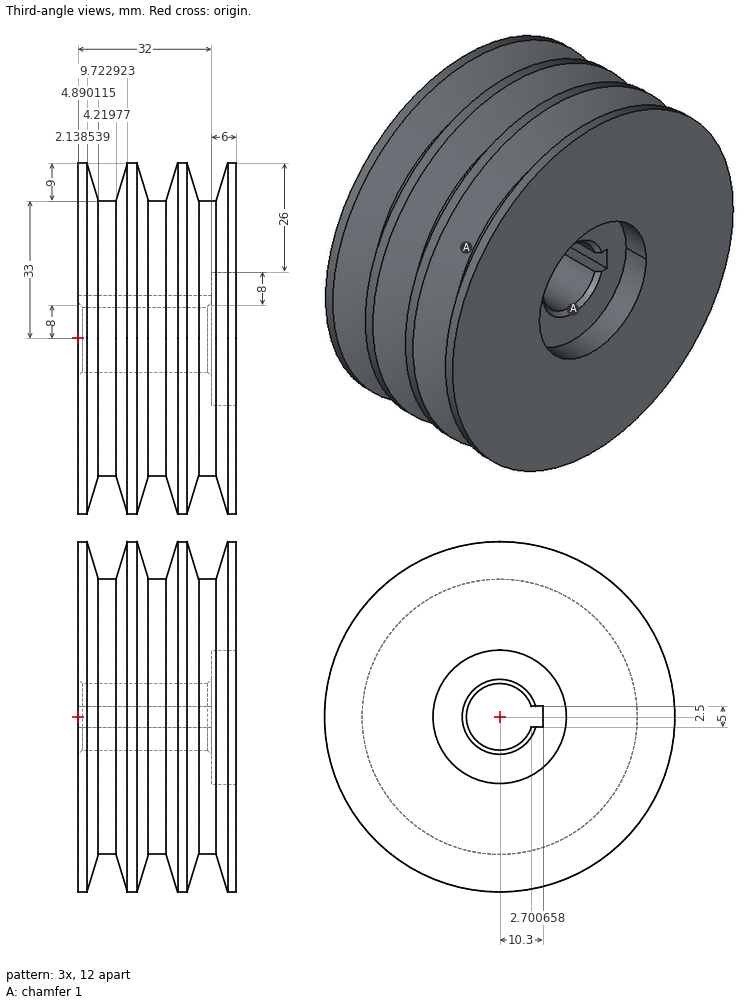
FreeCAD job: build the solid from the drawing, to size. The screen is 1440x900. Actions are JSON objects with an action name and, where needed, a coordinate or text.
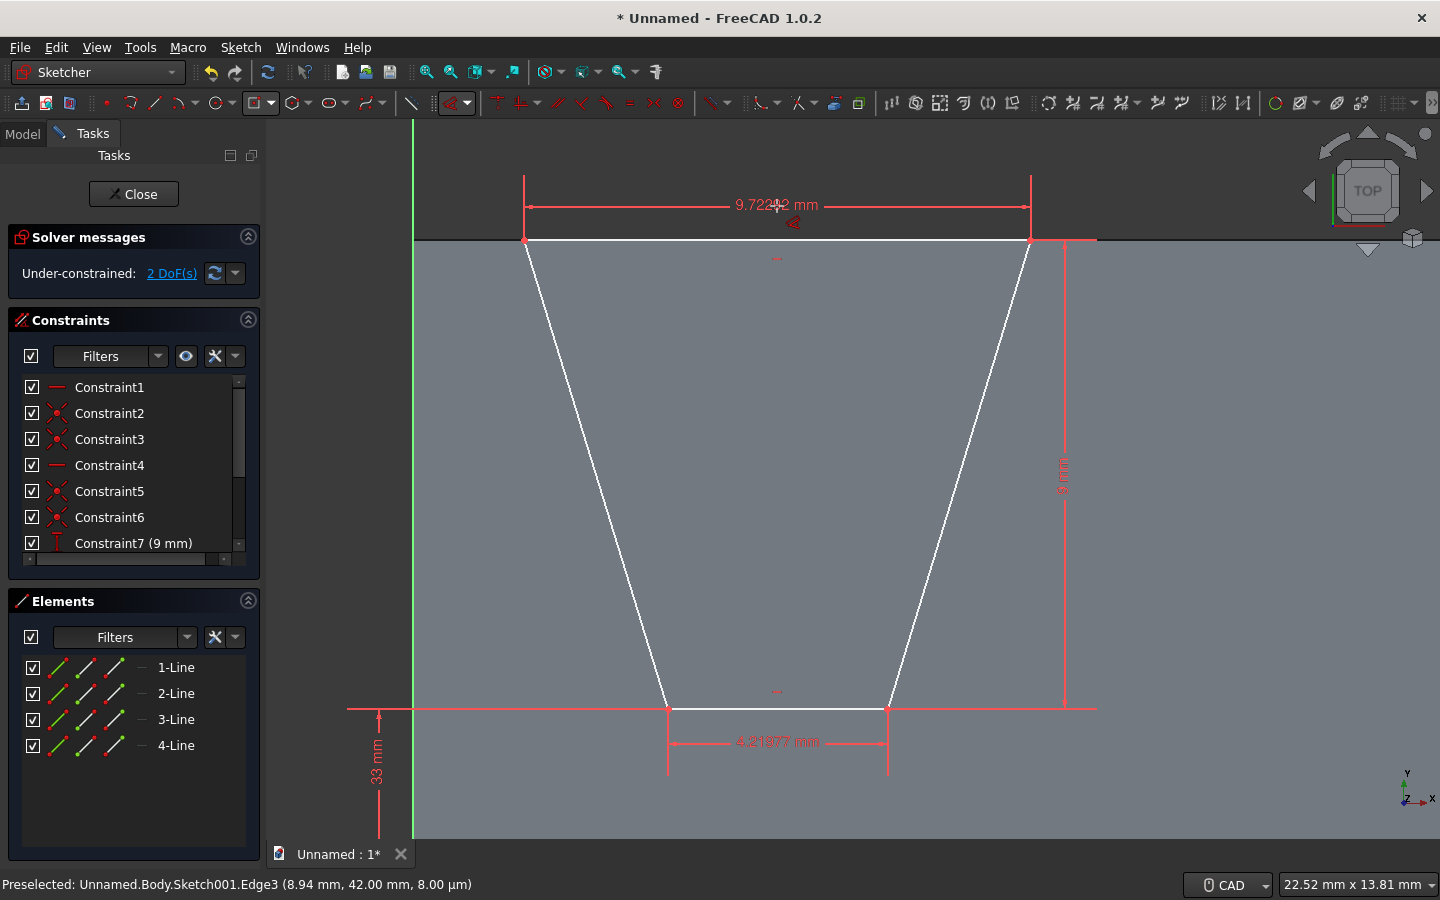
{"action": "left_click", "coordinate": [668, 709]}
{"action": "left_click", "coordinate": [540, 675]}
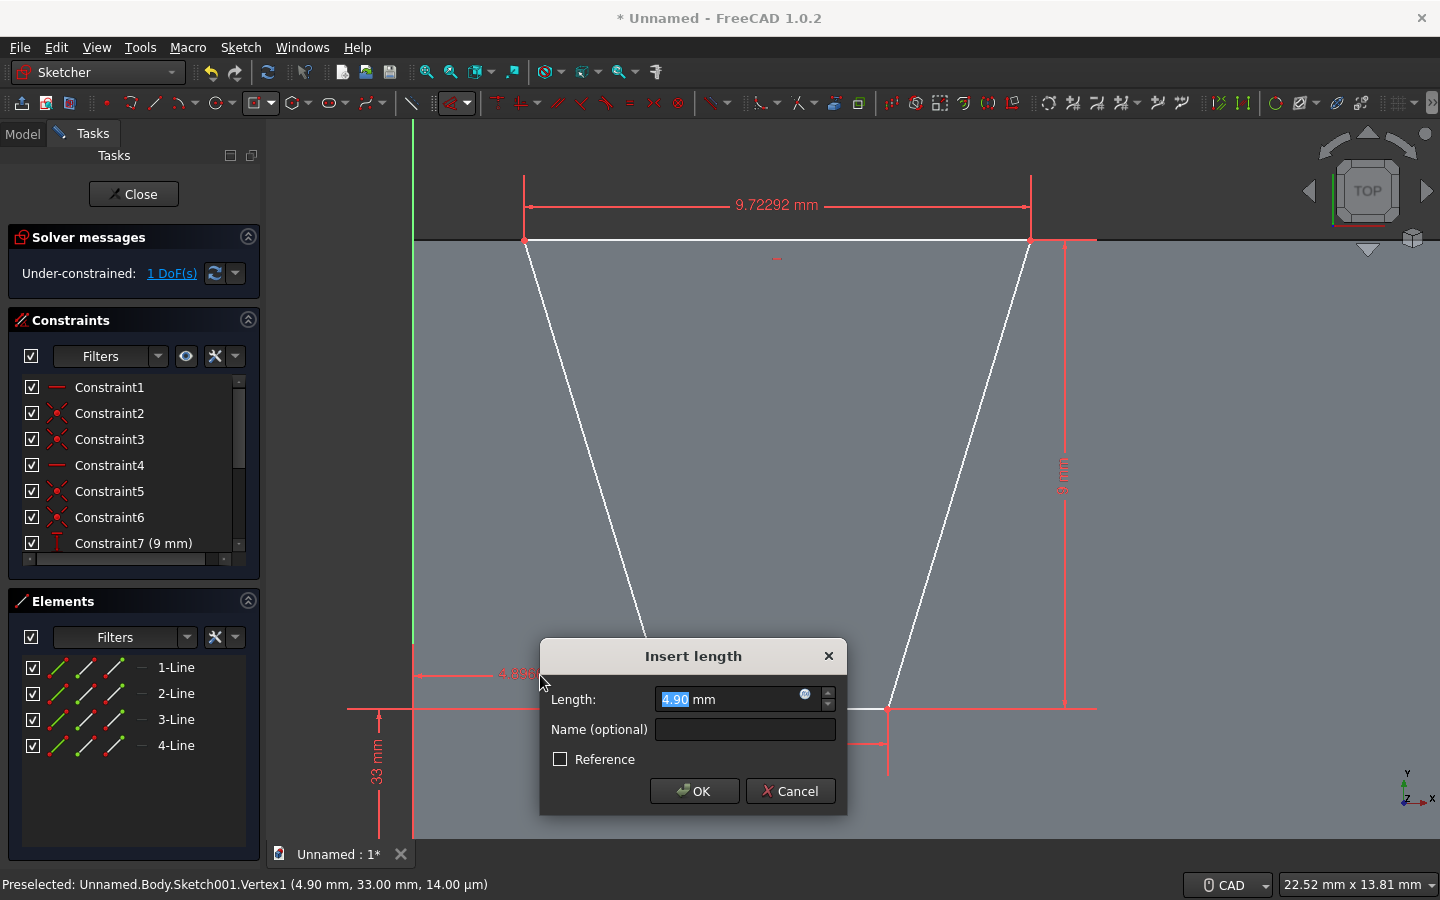
{"action": "type", "text": "4.890115"}
{"action": "key", "text": "Return"}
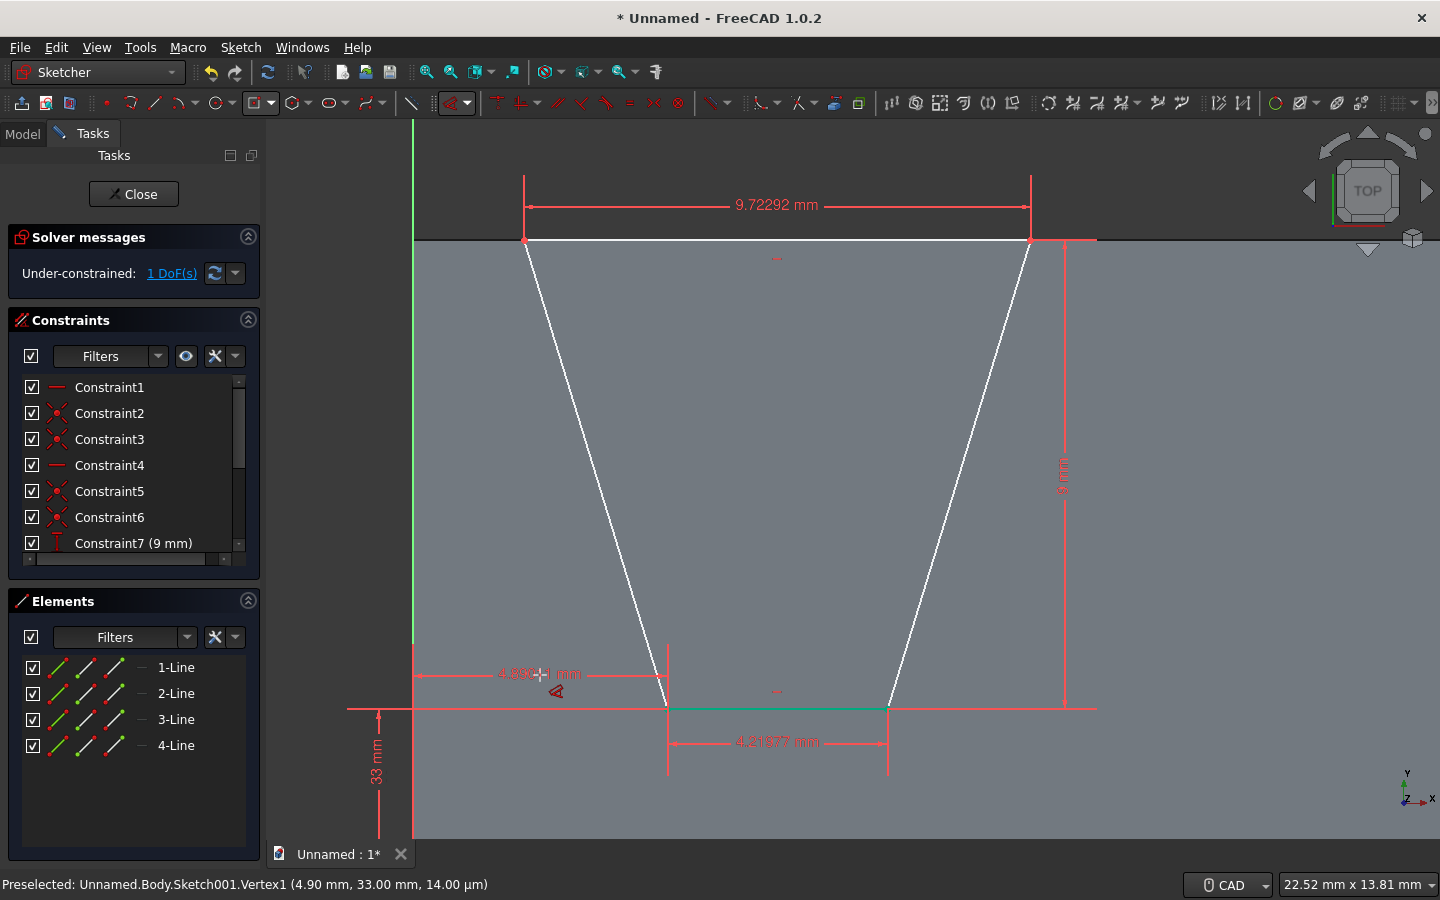
{"action": "left_click", "coordinate": [524, 240]}
{"action": "left_click", "coordinate": [468, 206]}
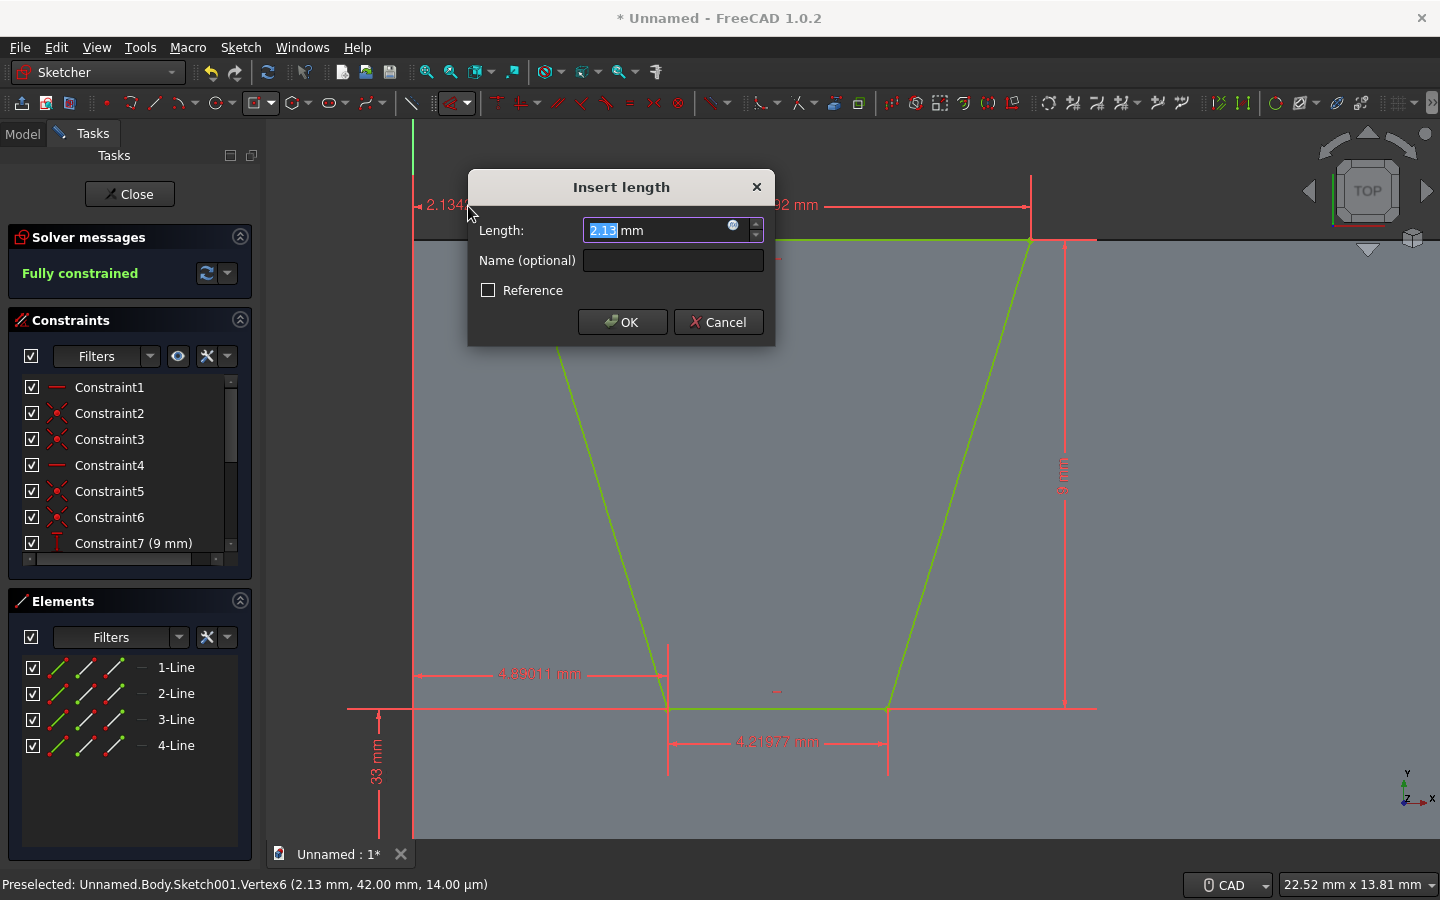
{"action": "type", "text": "2.138539"}
{"action": "key", "text": "Return"}
{"action": "key", "text": "Escape"}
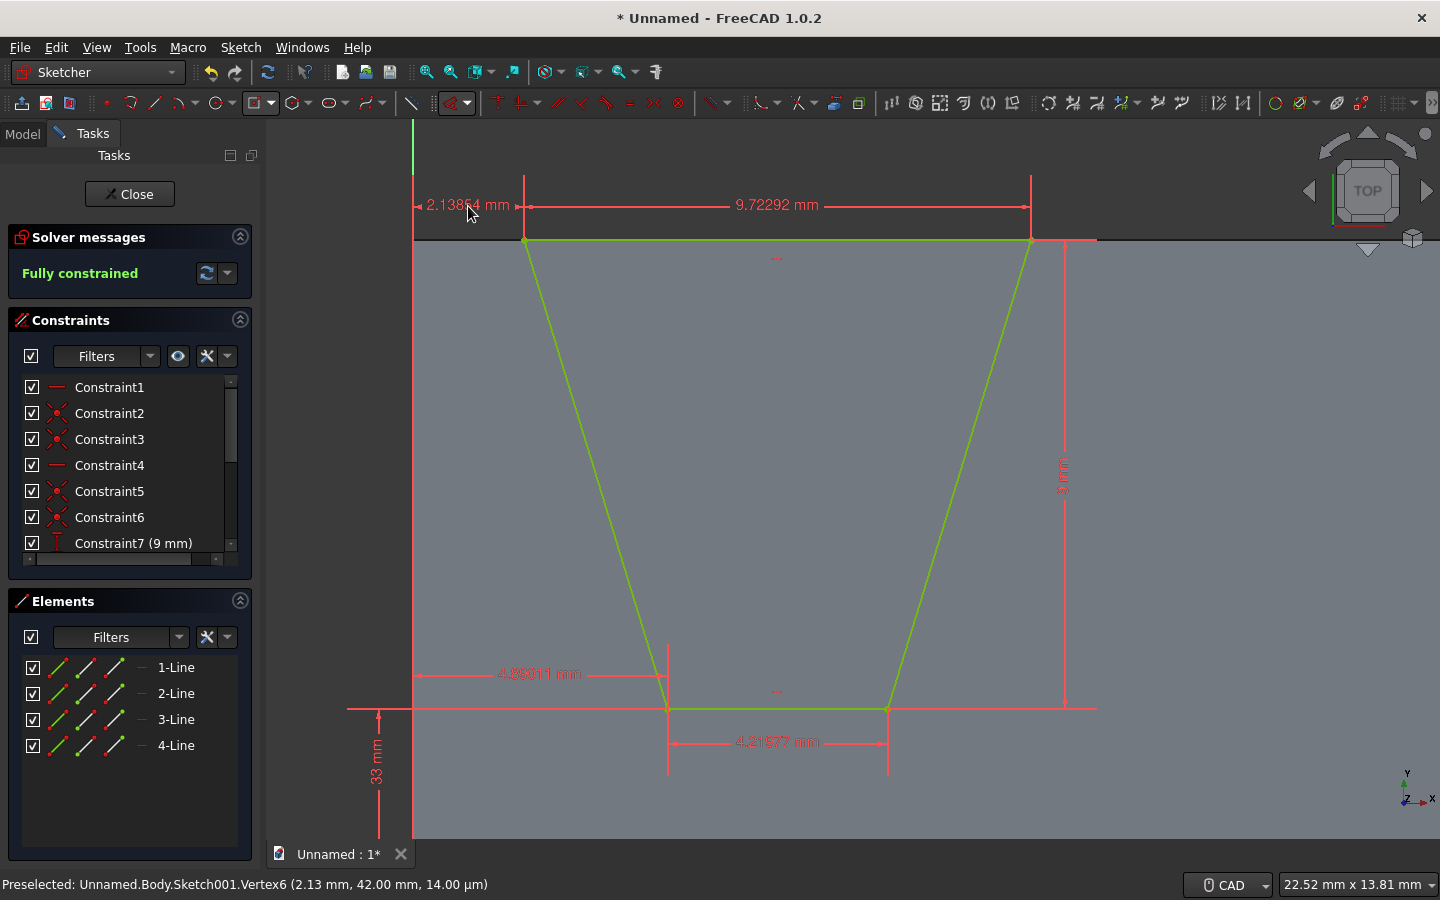
{"action": "left_click", "coordinate": [130, 194]}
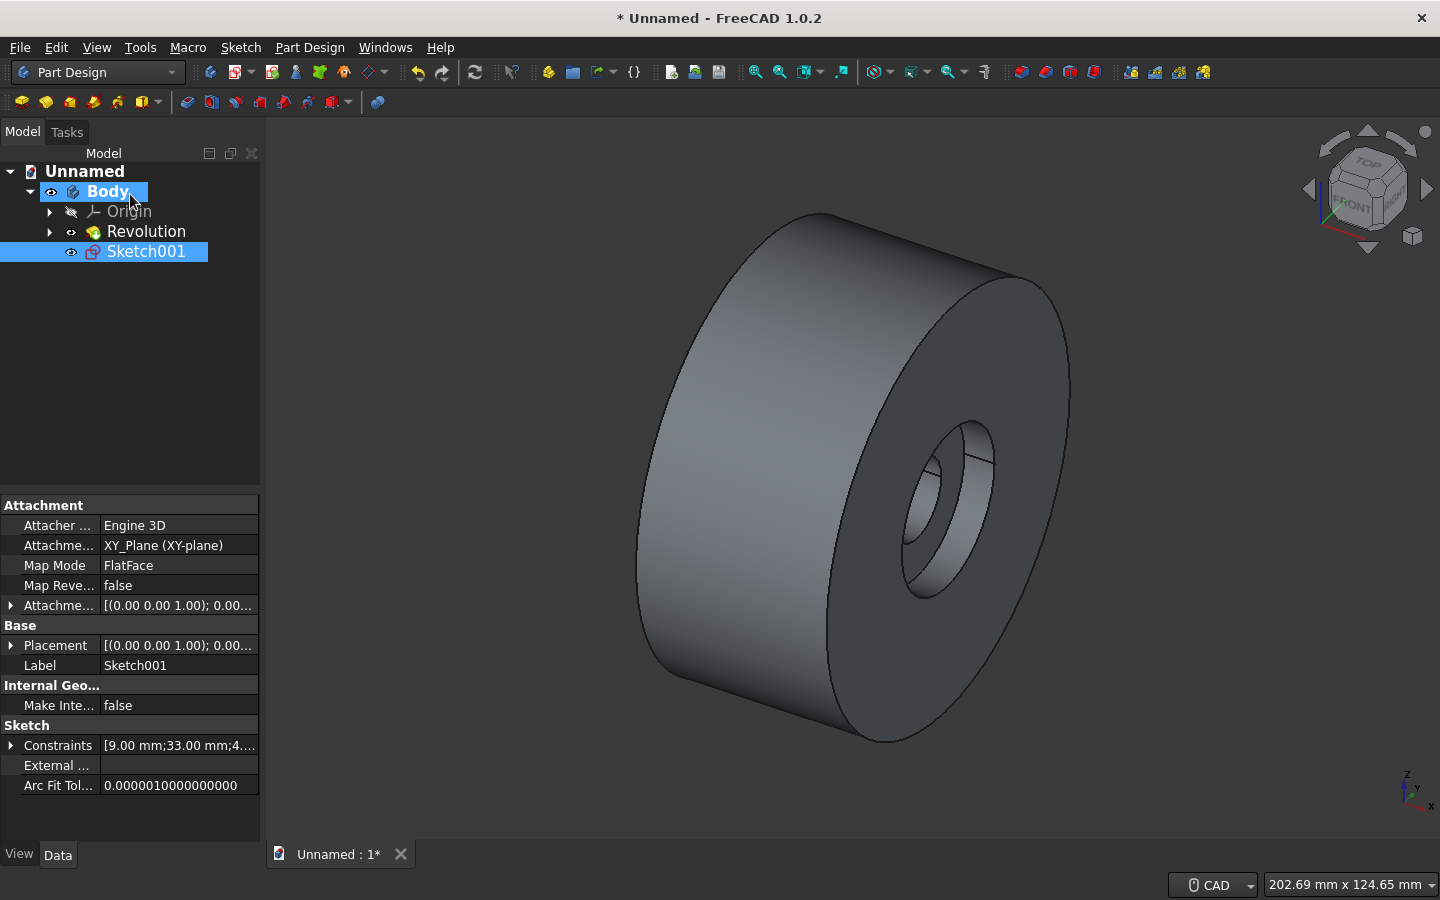
{"action": "left_click", "coordinate": [236, 102]}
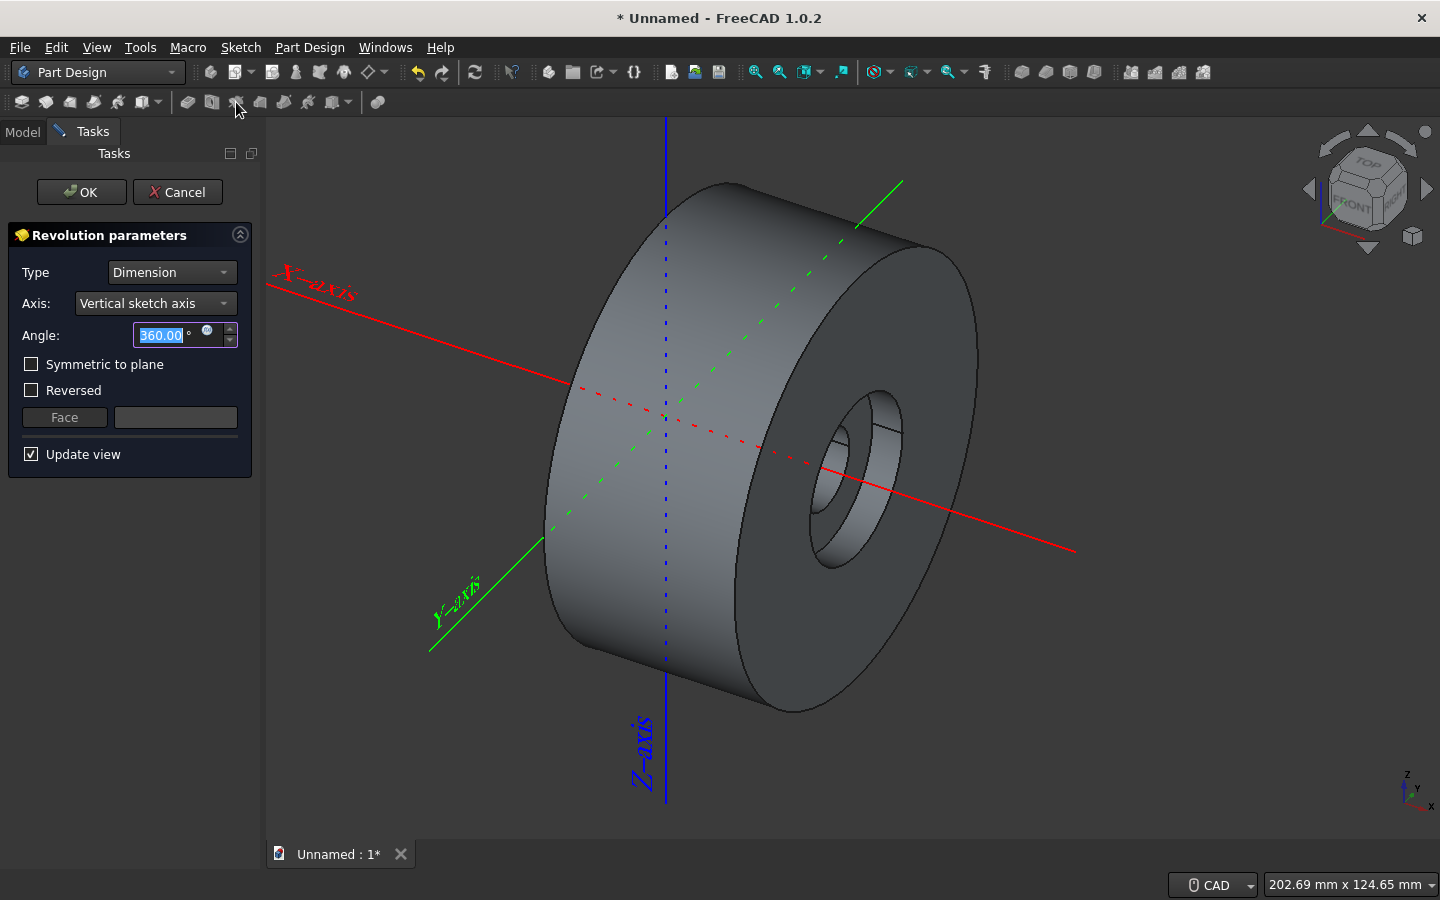
{"action": "left_click", "coordinate": [156, 304]}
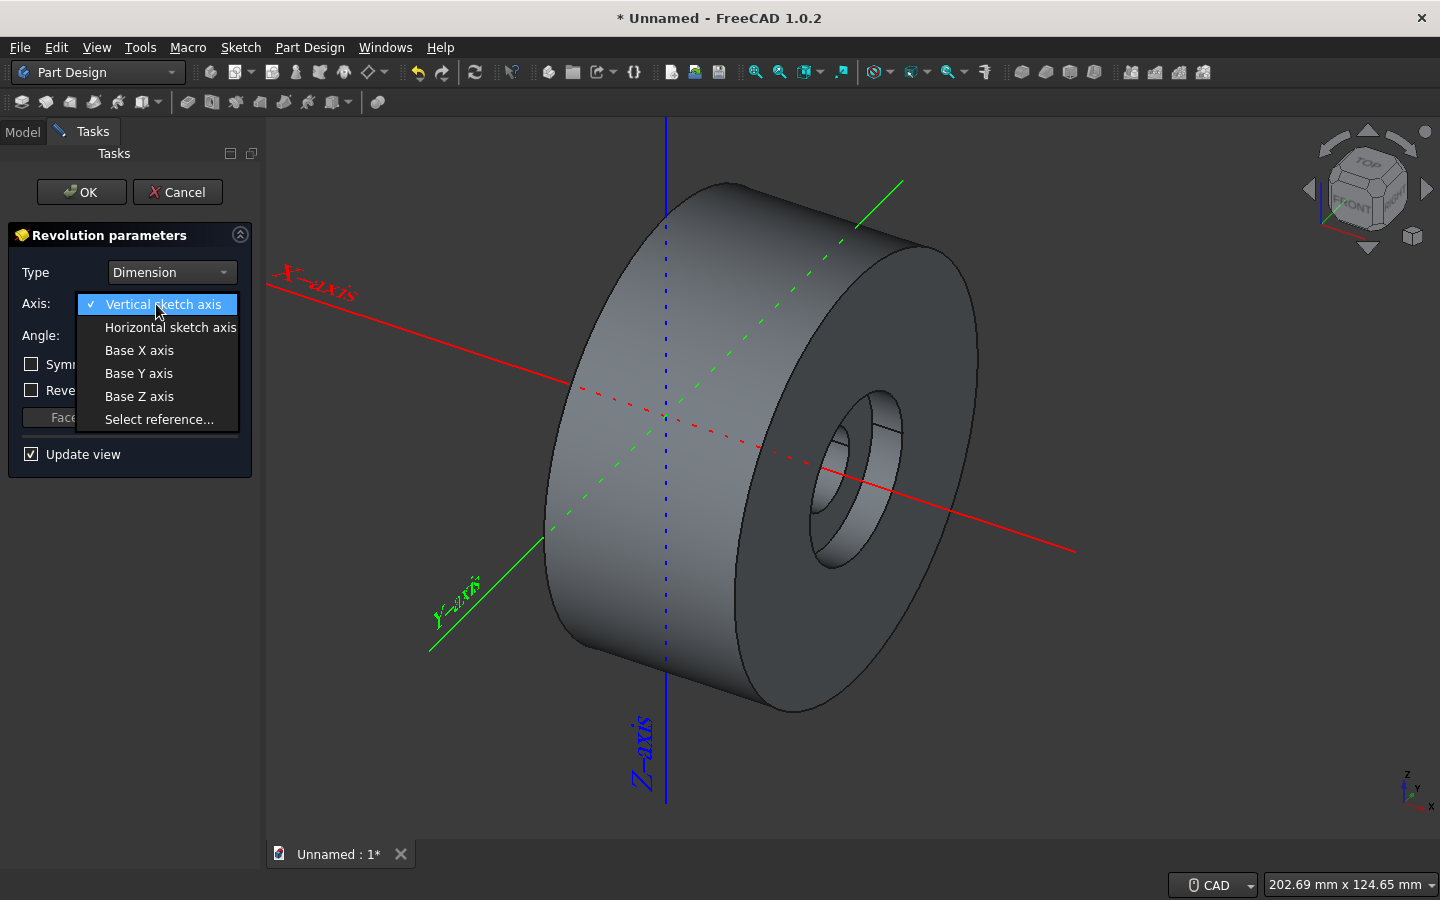
{"action": "left_click", "coordinate": [156, 328]}